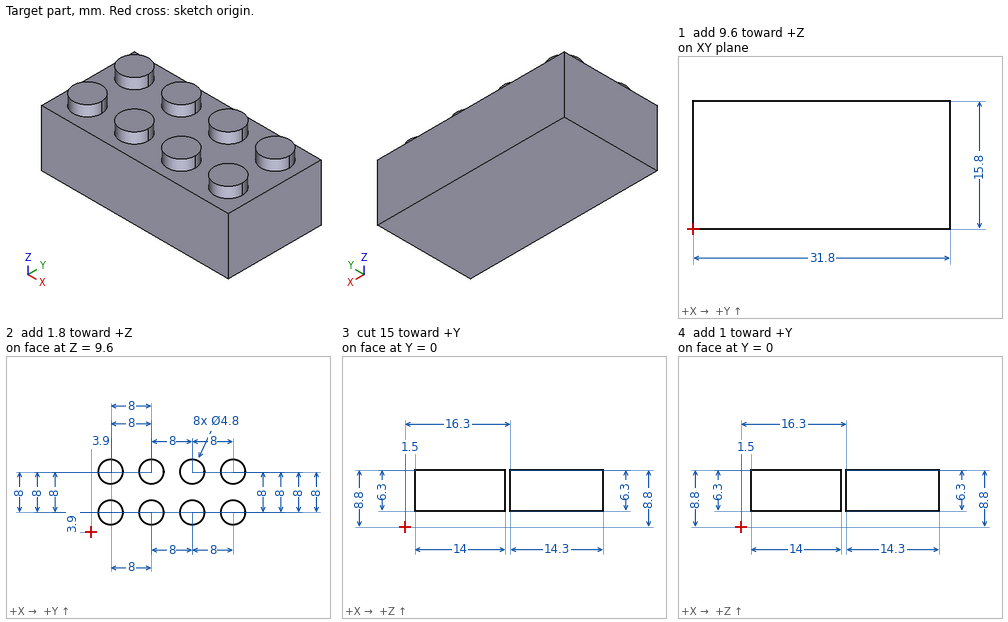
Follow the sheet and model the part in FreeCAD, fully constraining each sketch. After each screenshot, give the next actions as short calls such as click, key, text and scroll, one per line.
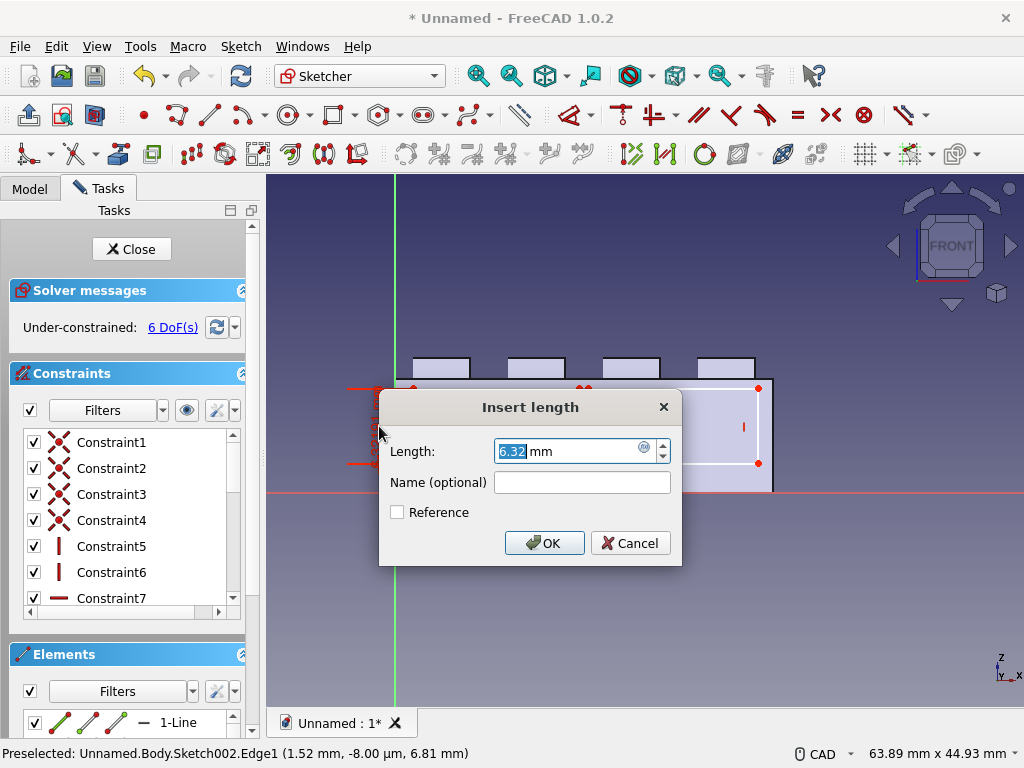
text(6.3)
key(Return)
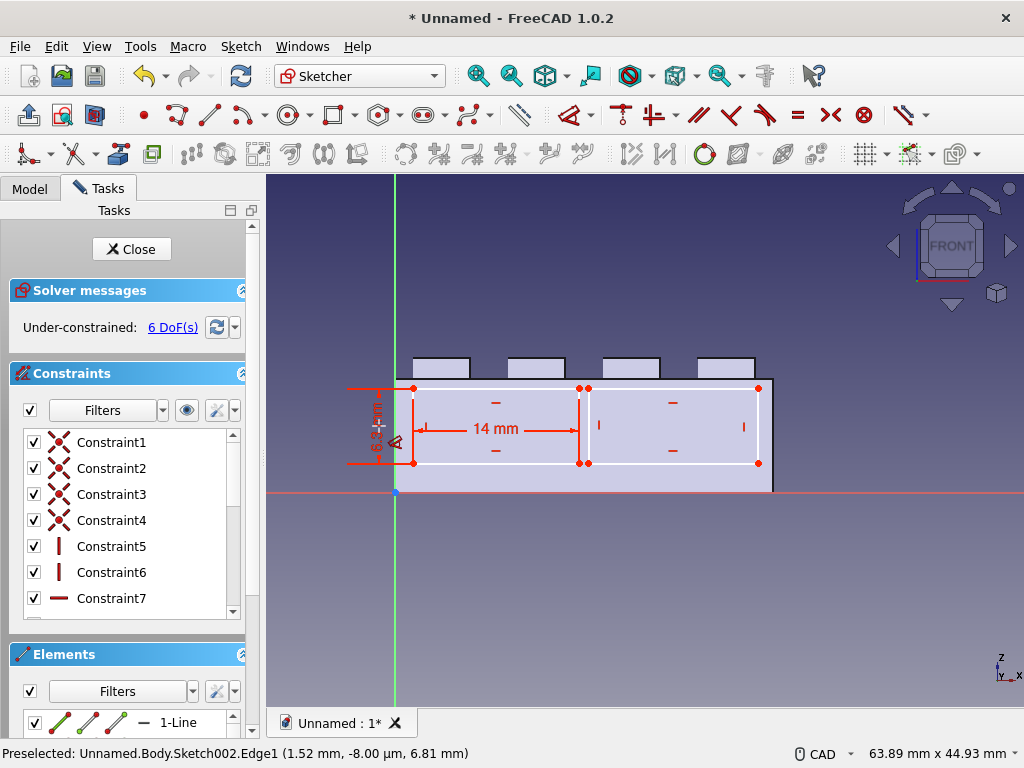
scroll(589, 411, up, 3)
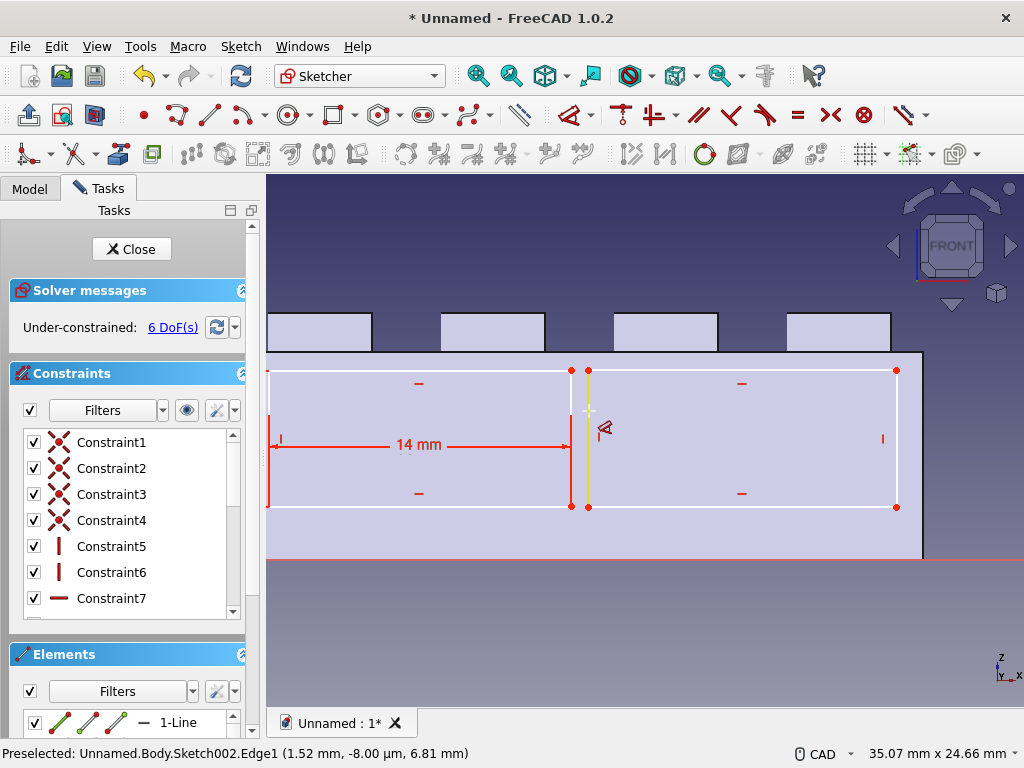
click(588, 411)
click(622, 439)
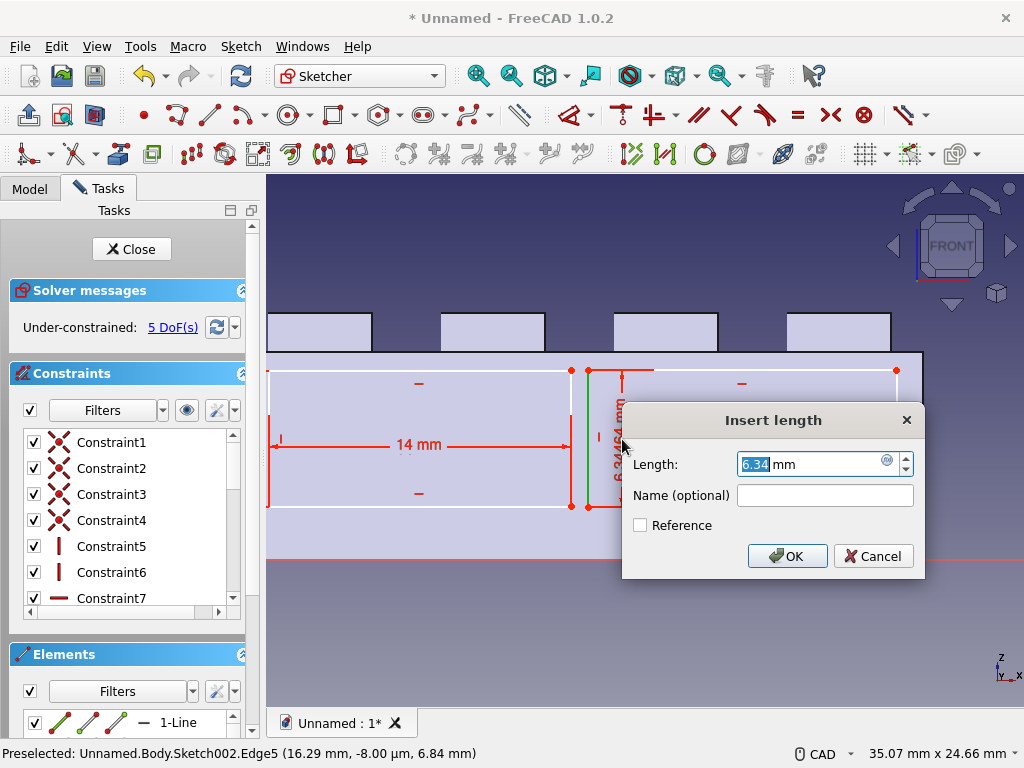
text(6.3)
key(Return)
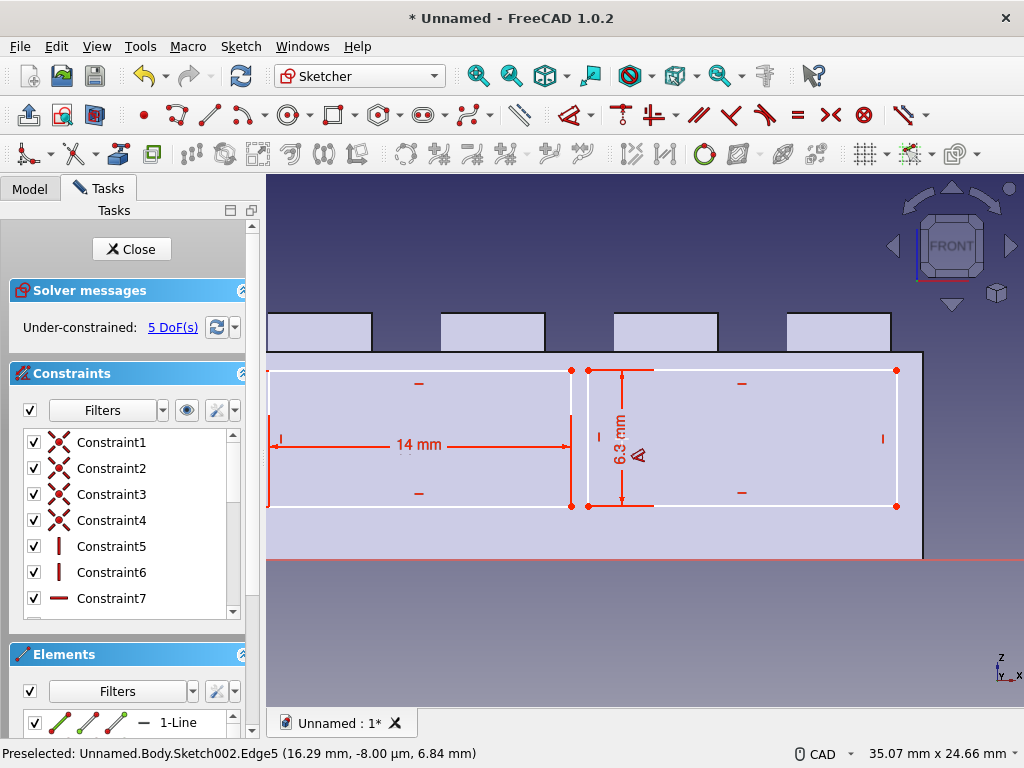
click(681, 506)
click(724, 540)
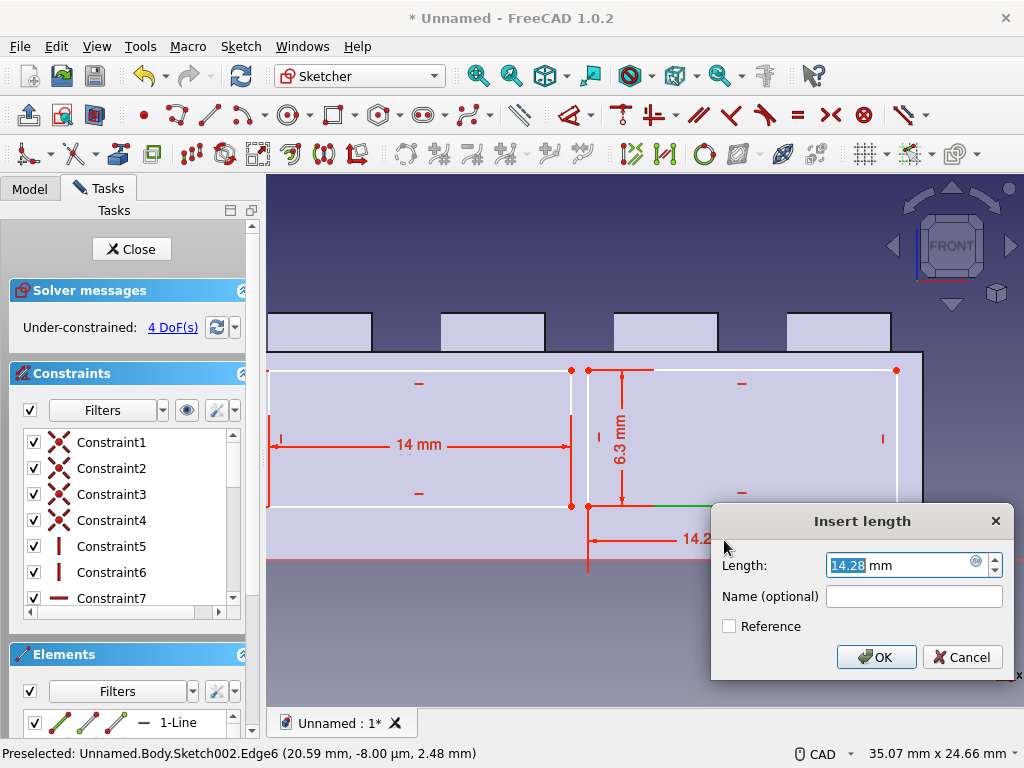
text(14.3)
key(Return)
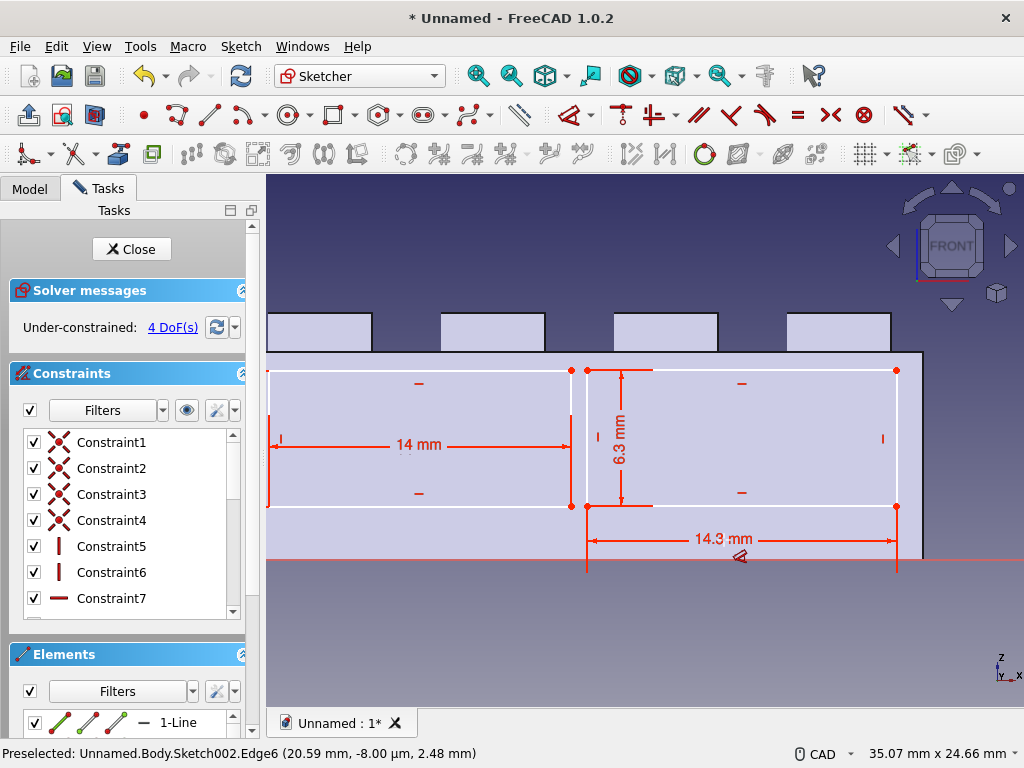
scroll(589, 411, down, 3)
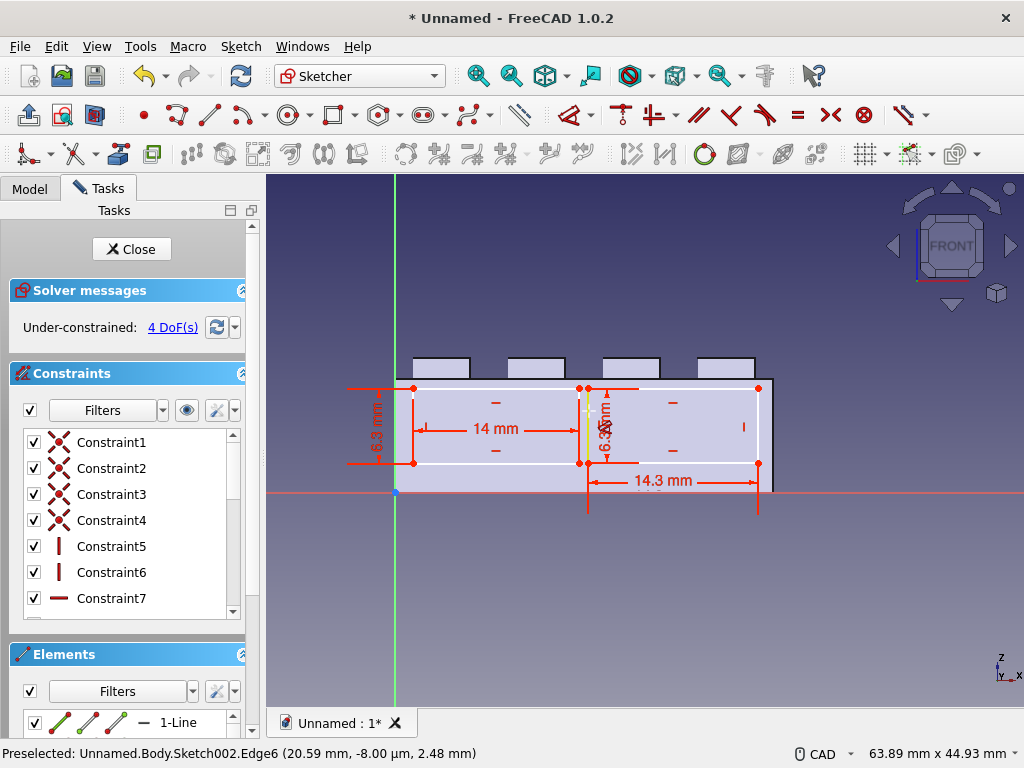
scroll(413, 389, up, 5)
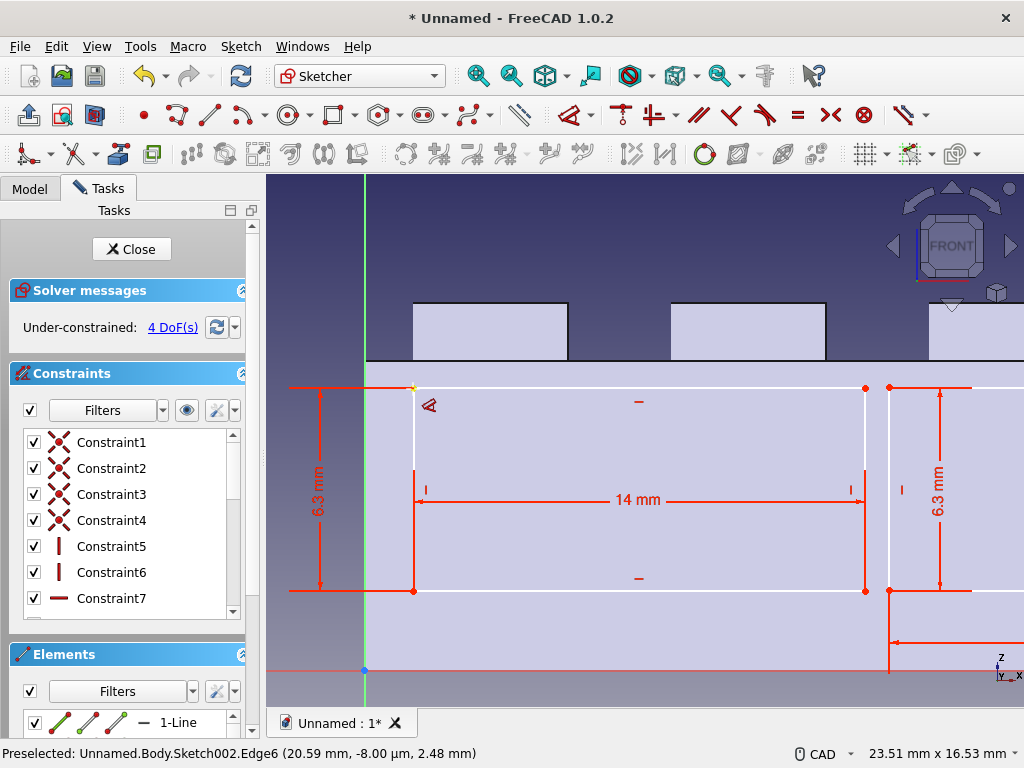
click(414, 388)
click(389, 354)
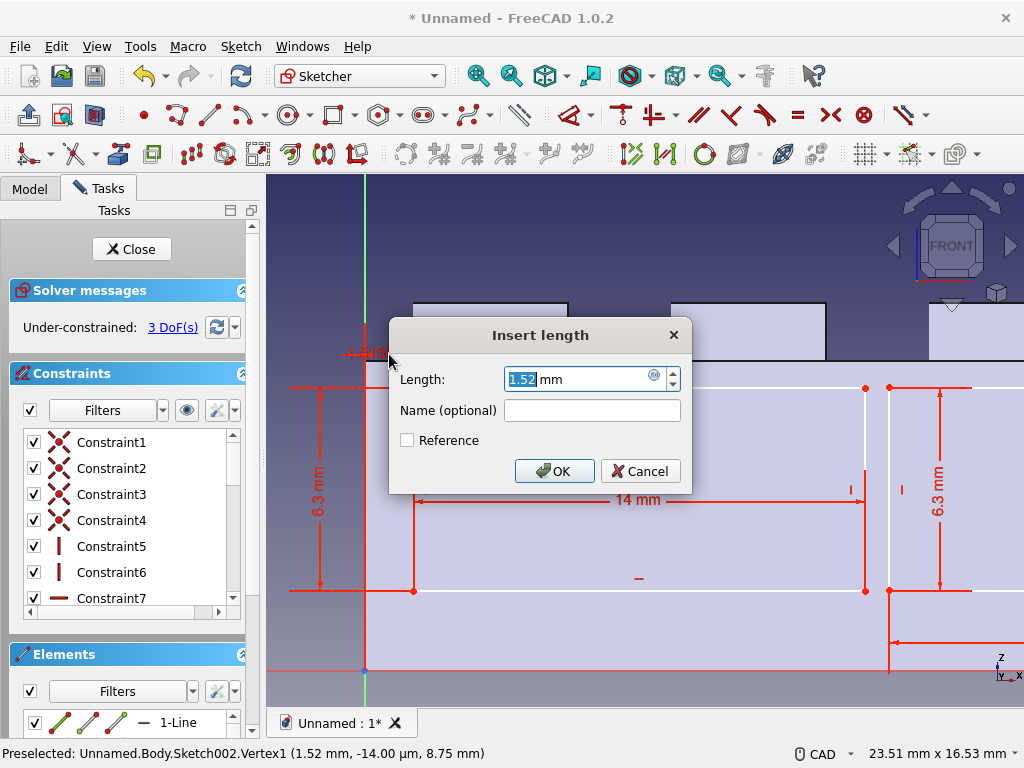
text(1.5)
key(Return)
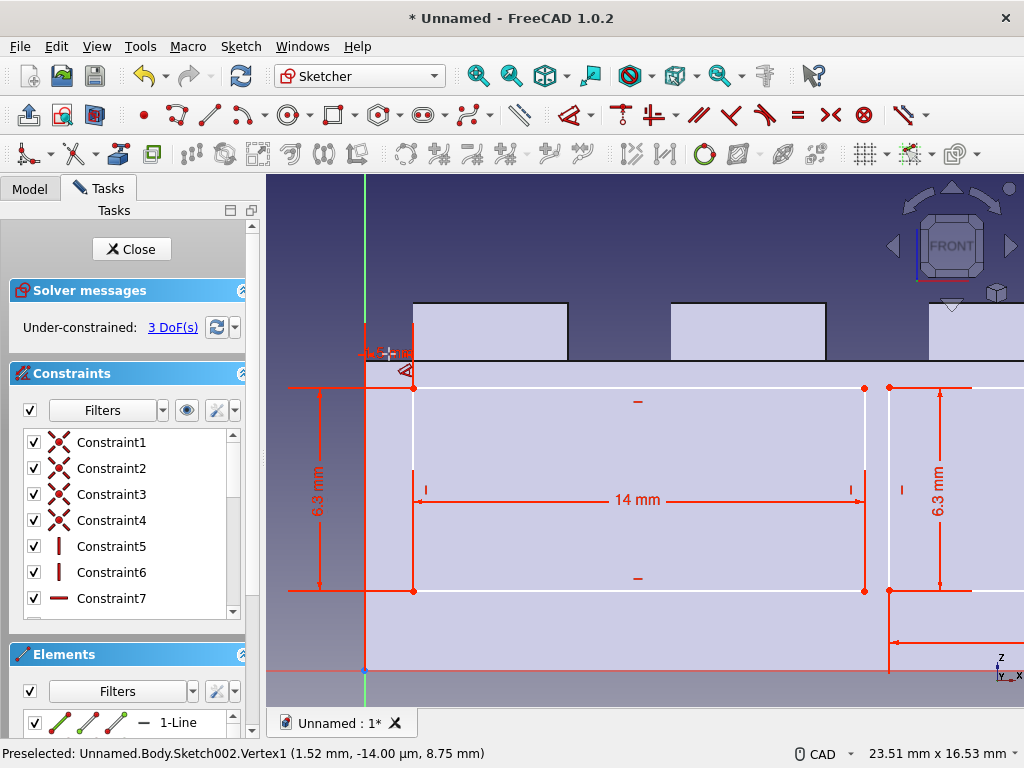
click(413, 388)
click(331, 529)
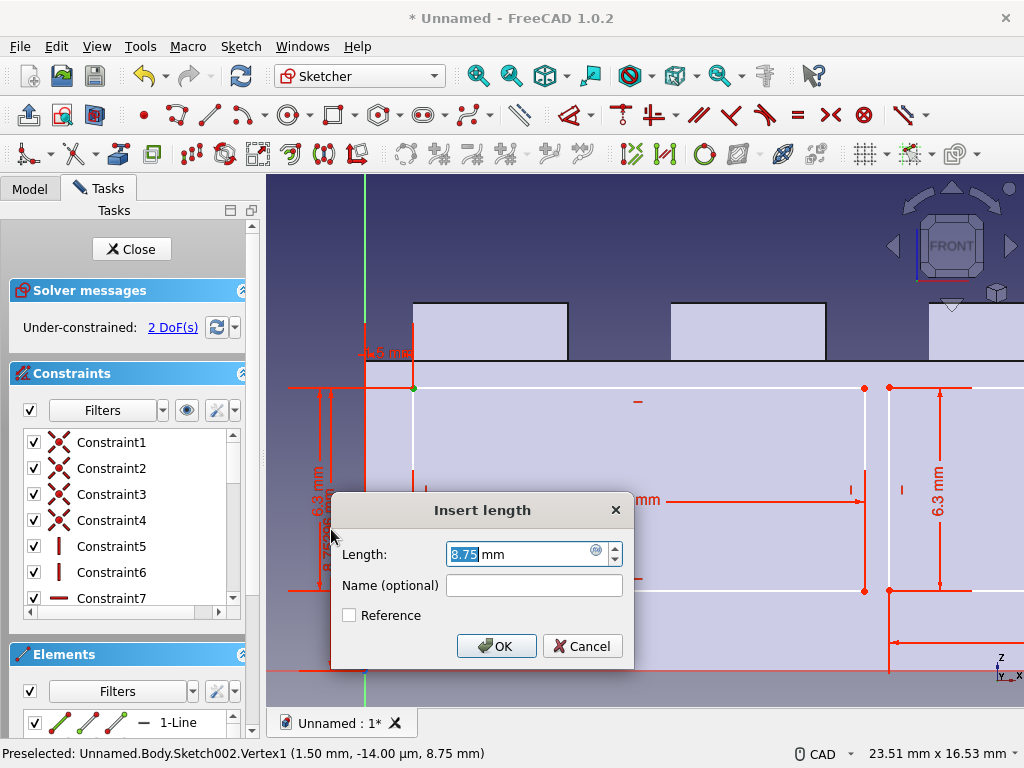
text(8.8)
key(Return)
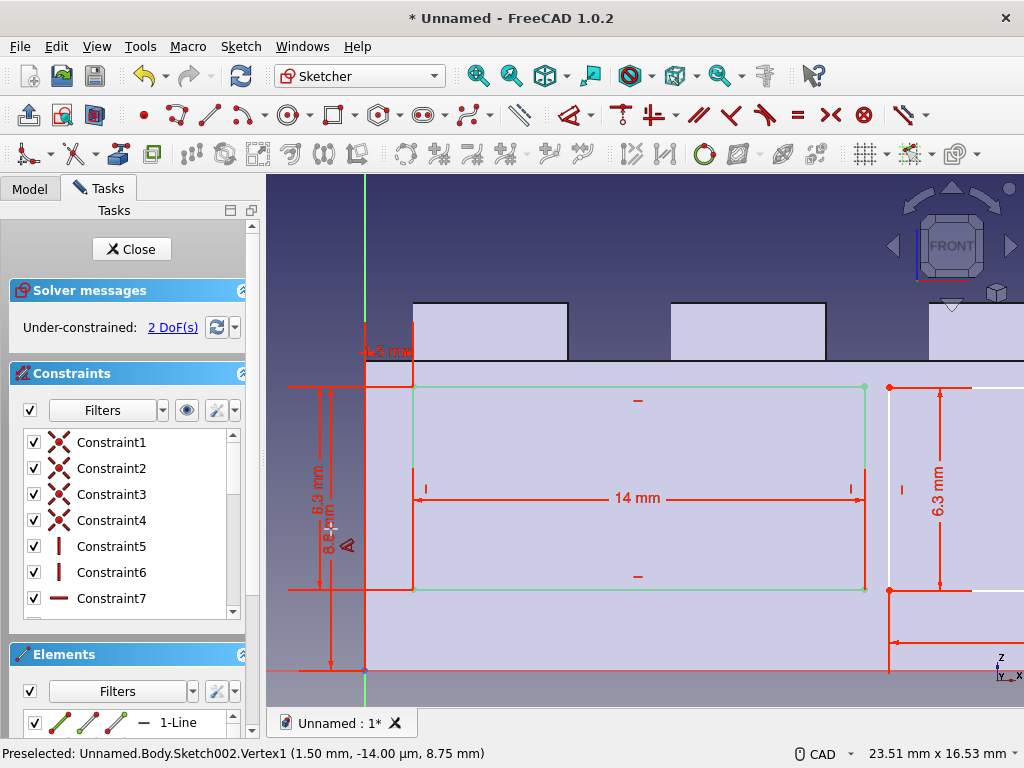
scroll(413, 389, down, 5)